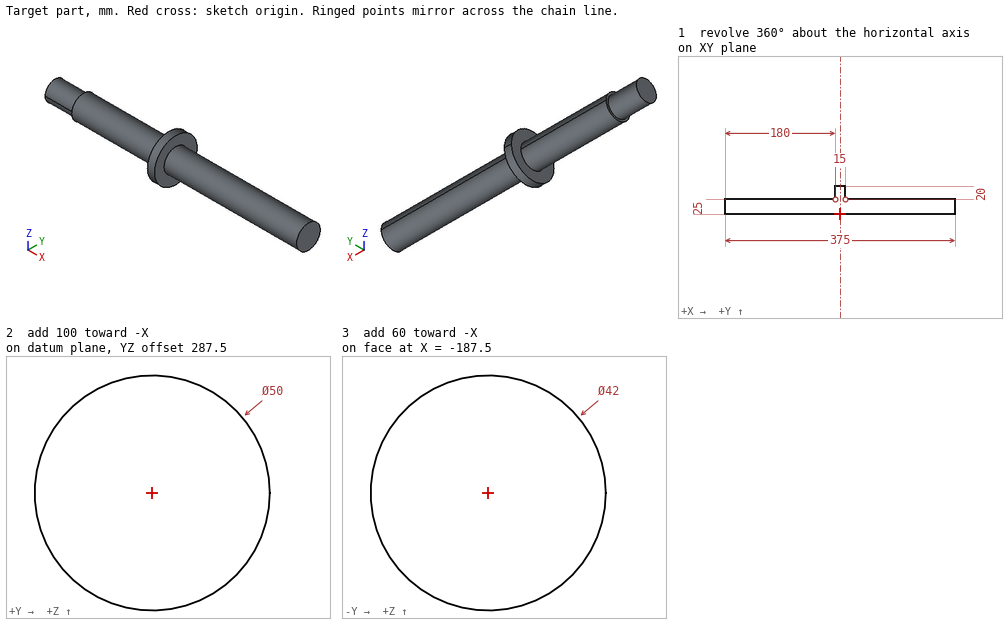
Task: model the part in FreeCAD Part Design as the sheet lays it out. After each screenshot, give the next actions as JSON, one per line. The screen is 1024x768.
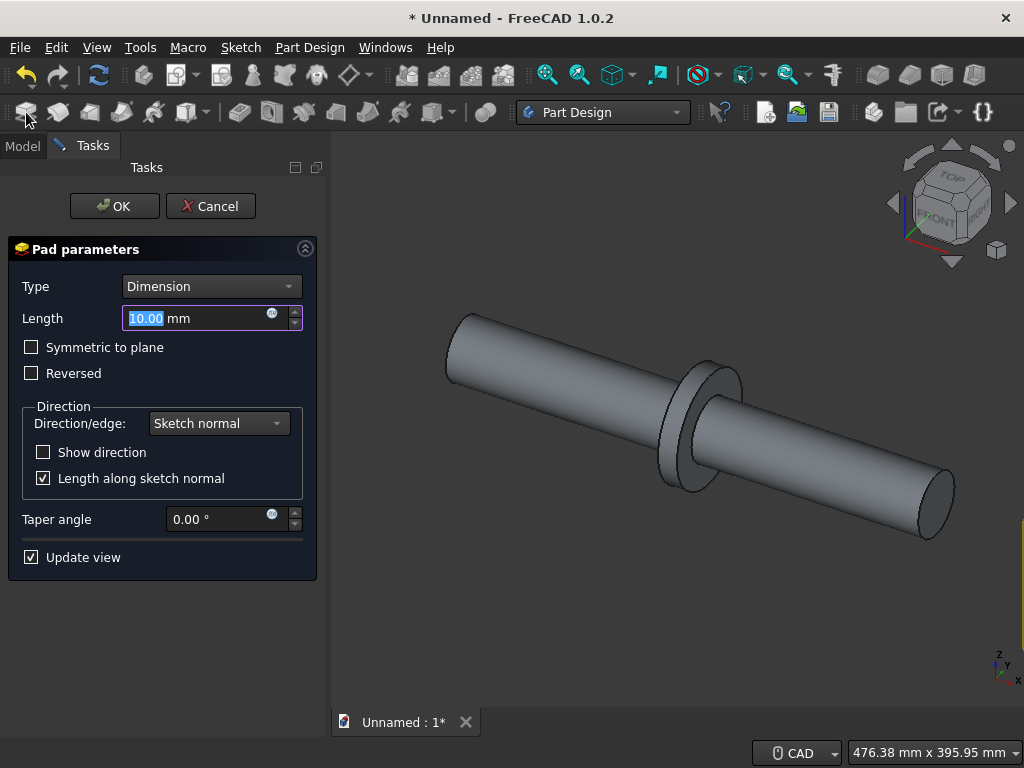
{"action": "type", "text": "100"}
{"action": "key", "text": "Tab"}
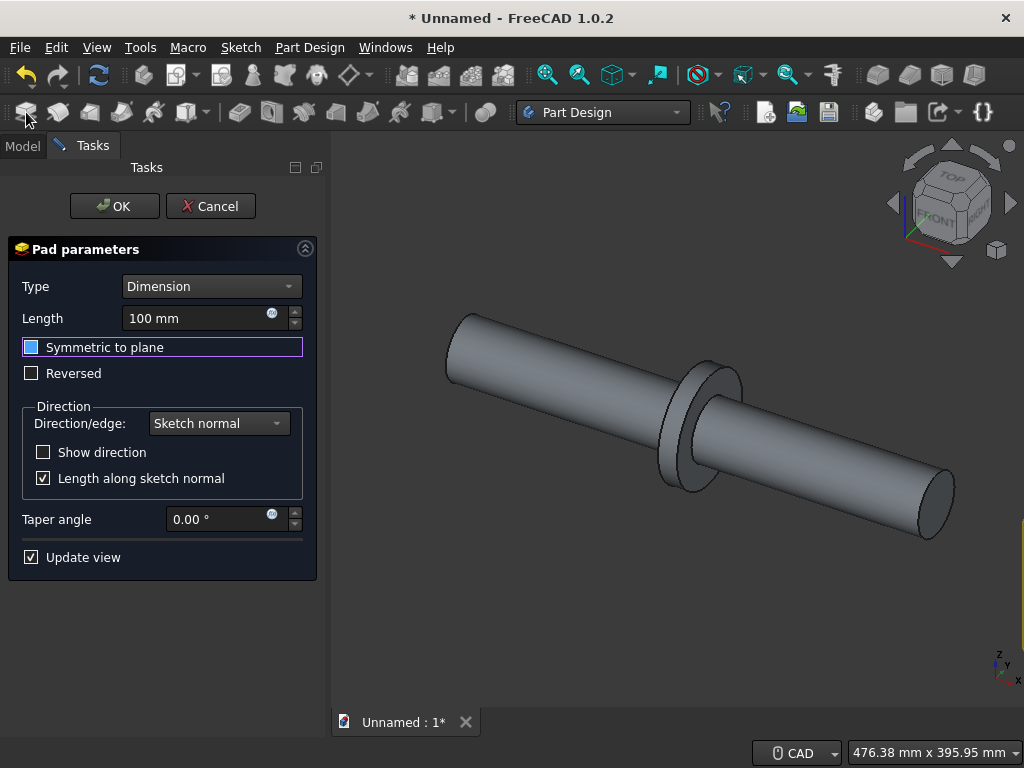
{"action": "left_click", "coordinate": [30, 373]}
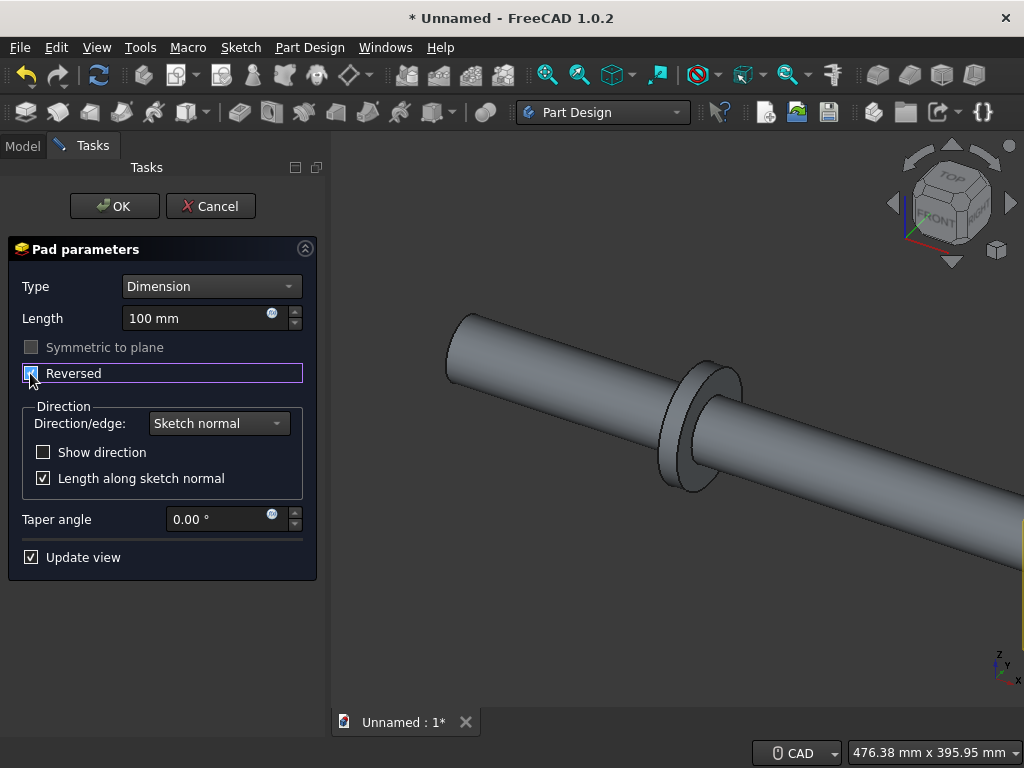
{"action": "left_click", "coordinate": [115, 206]}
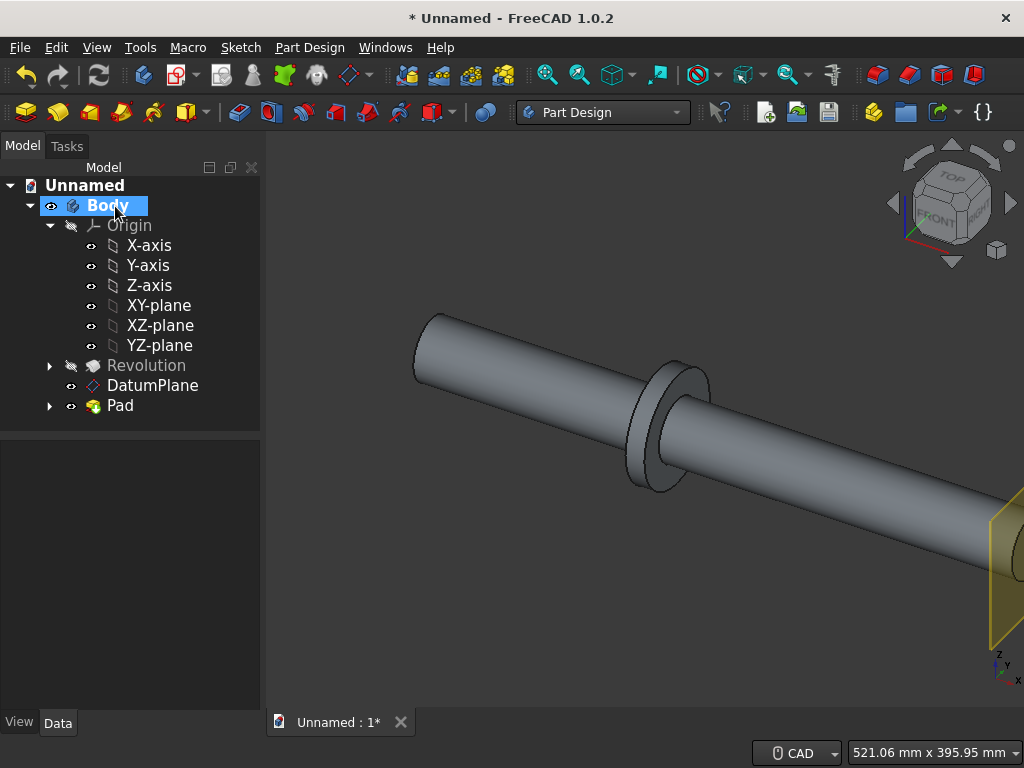
{"action": "left_click", "coordinate": [116, 386]}
{"action": "key", "text": "space"}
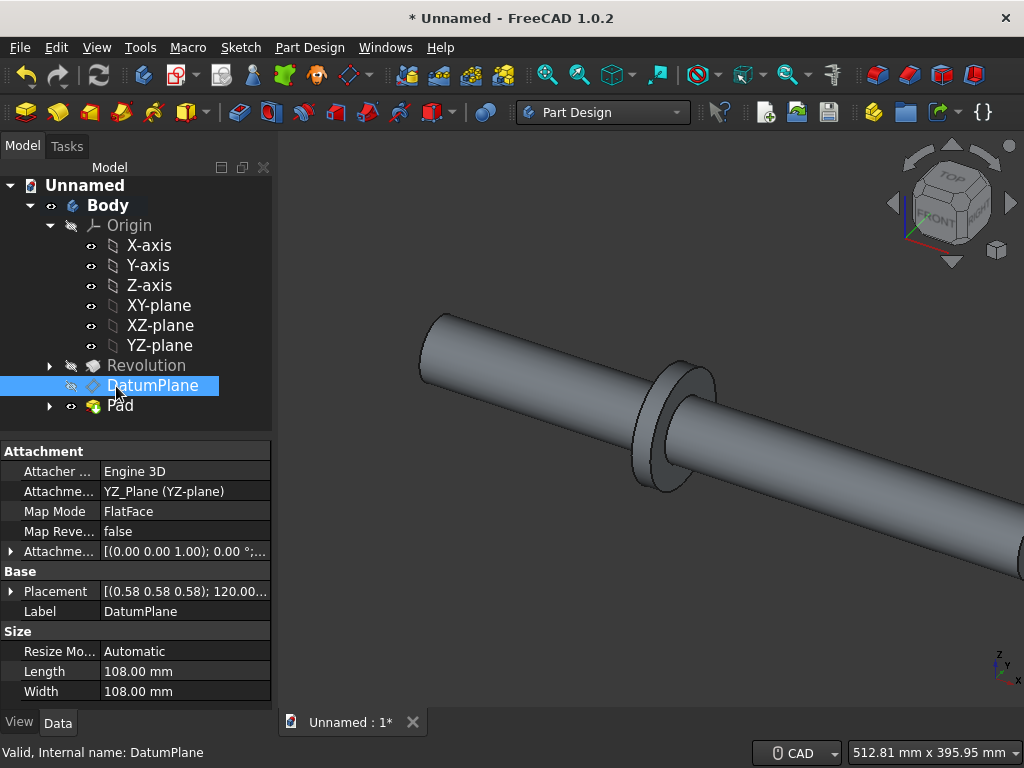
{"action": "left_click", "coordinate": [548, 76]}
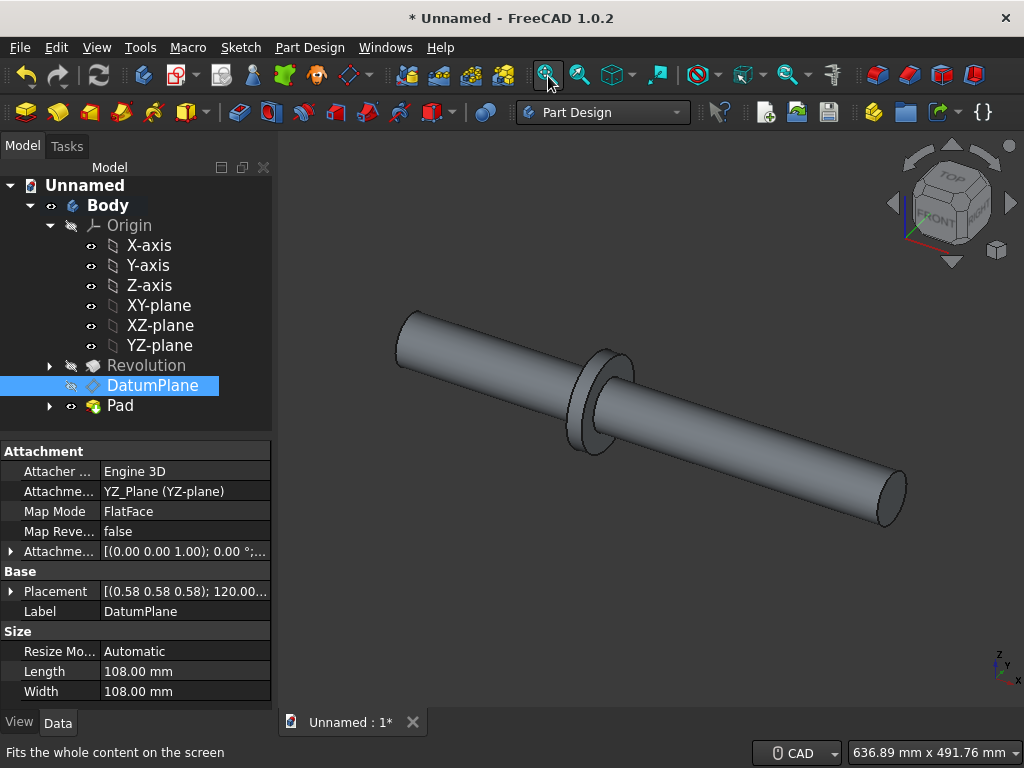
{"action": "key", "text": "6"}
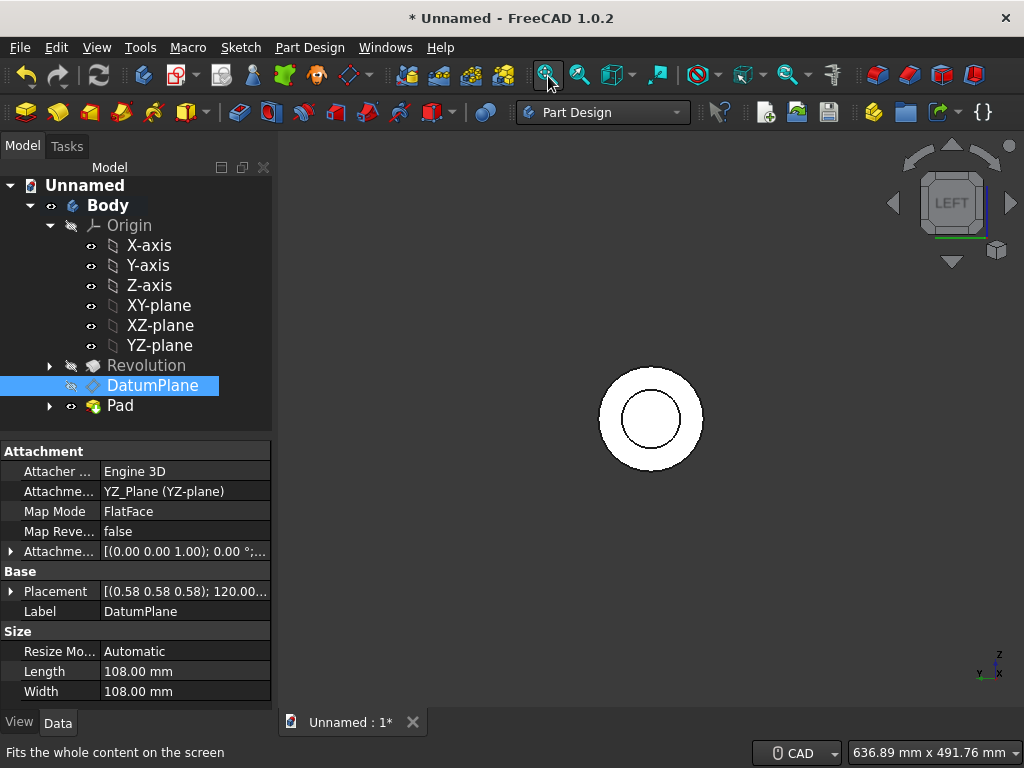
{"action": "key", "text": "v f"}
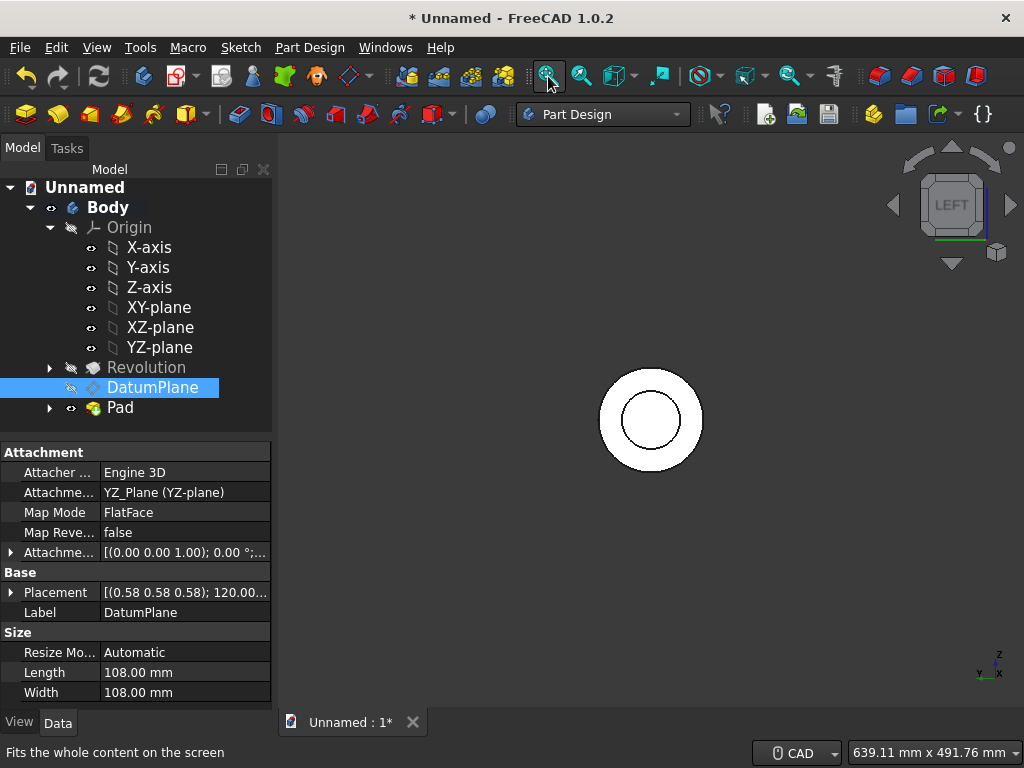
{"action": "left_click", "coordinate": [651, 419]}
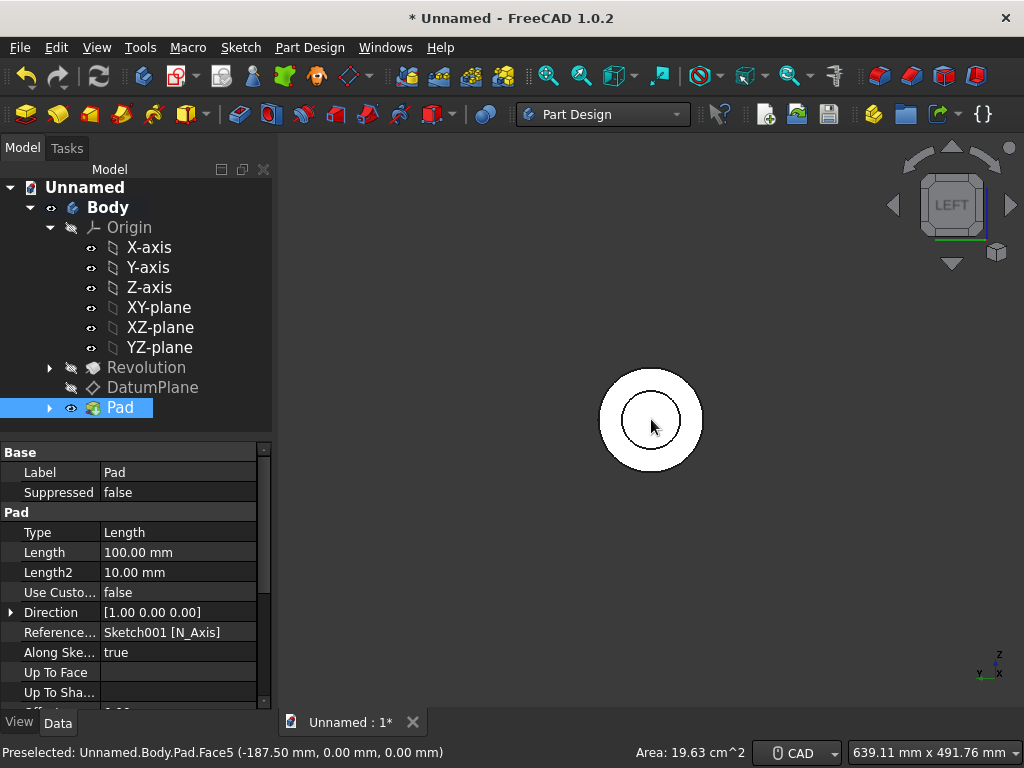
{"action": "left_click", "coordinate": [176, 76]}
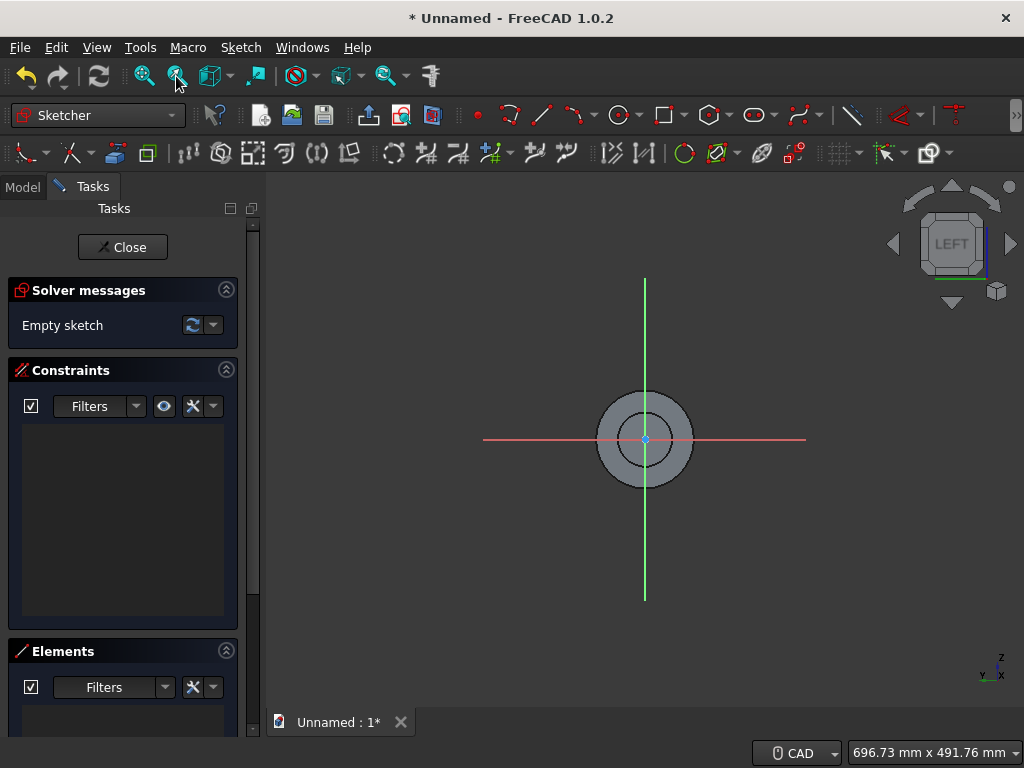
{"action": "scroll", "coordinate": [656, 440], "scroll_direction": "up", "scroll_amount": 10}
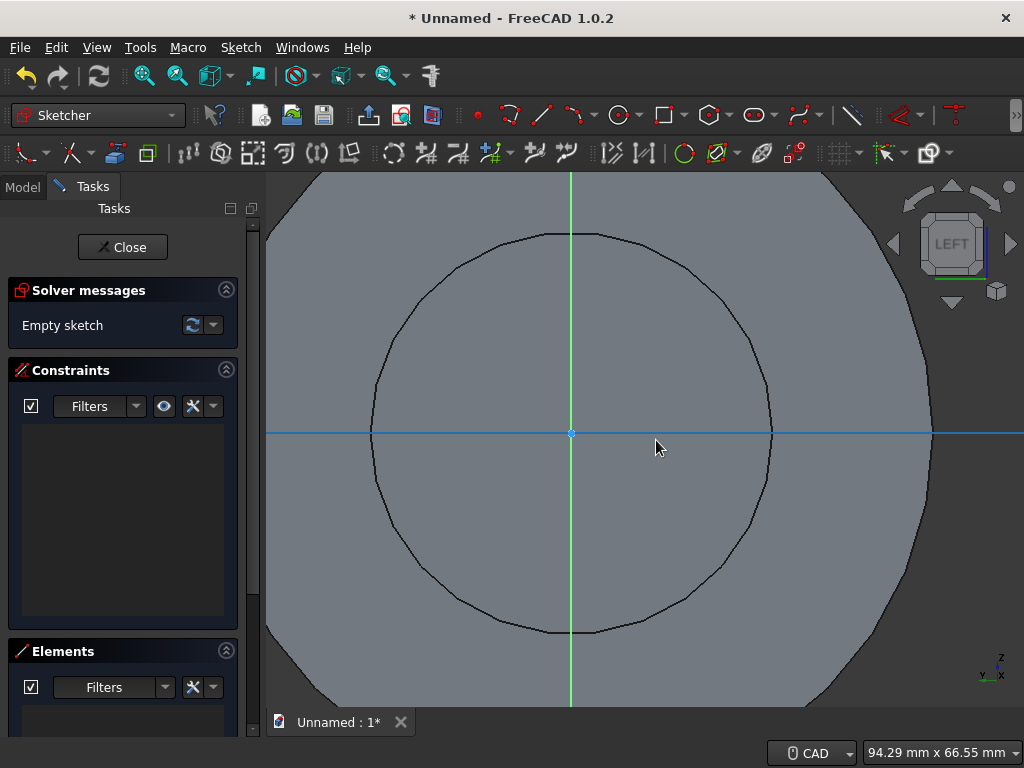
{"action": "left_click", "coordinate": [620, 116]}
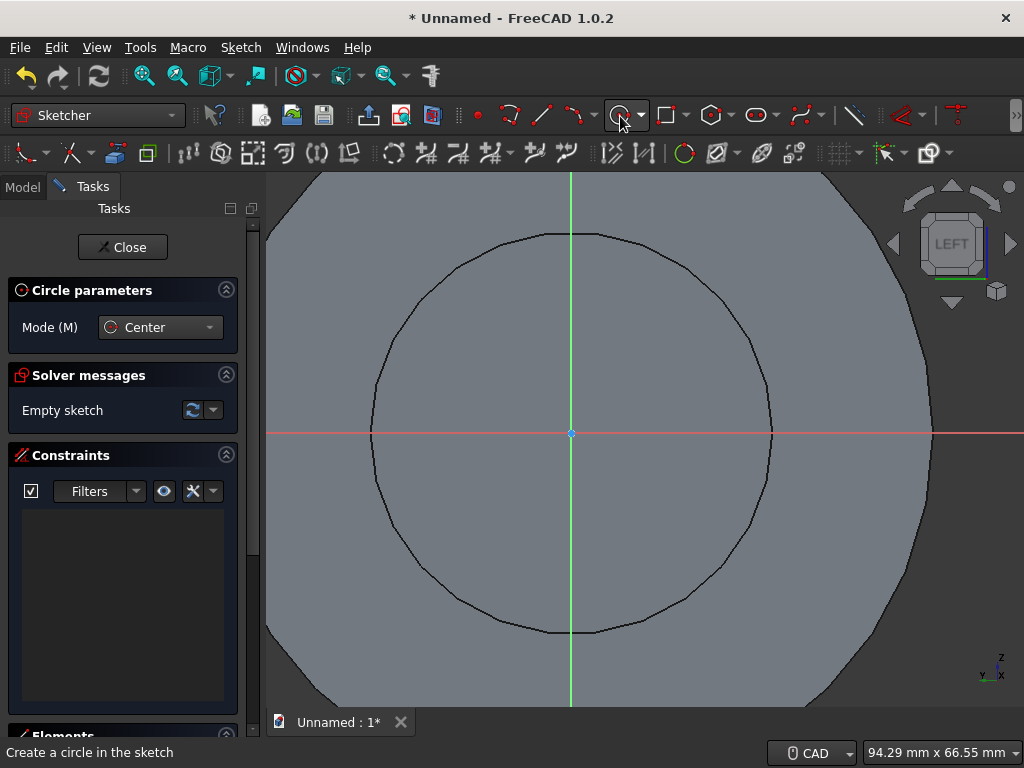
{"action": "left_click", "coordinate": [571, 433]}
{"action": "mouse_move", "coordinate": [691, 314]}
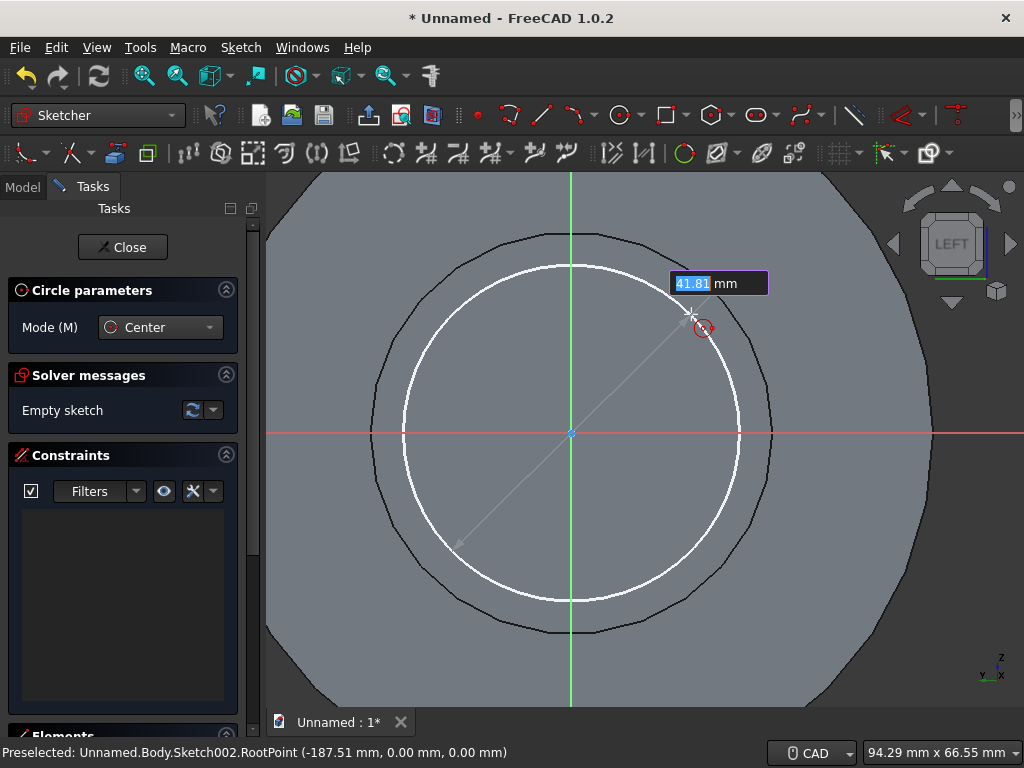
{"action": "type", "text": "42"}
{"action": "key", "text": "Return"}
{"action": "key", "text": "Escape"}